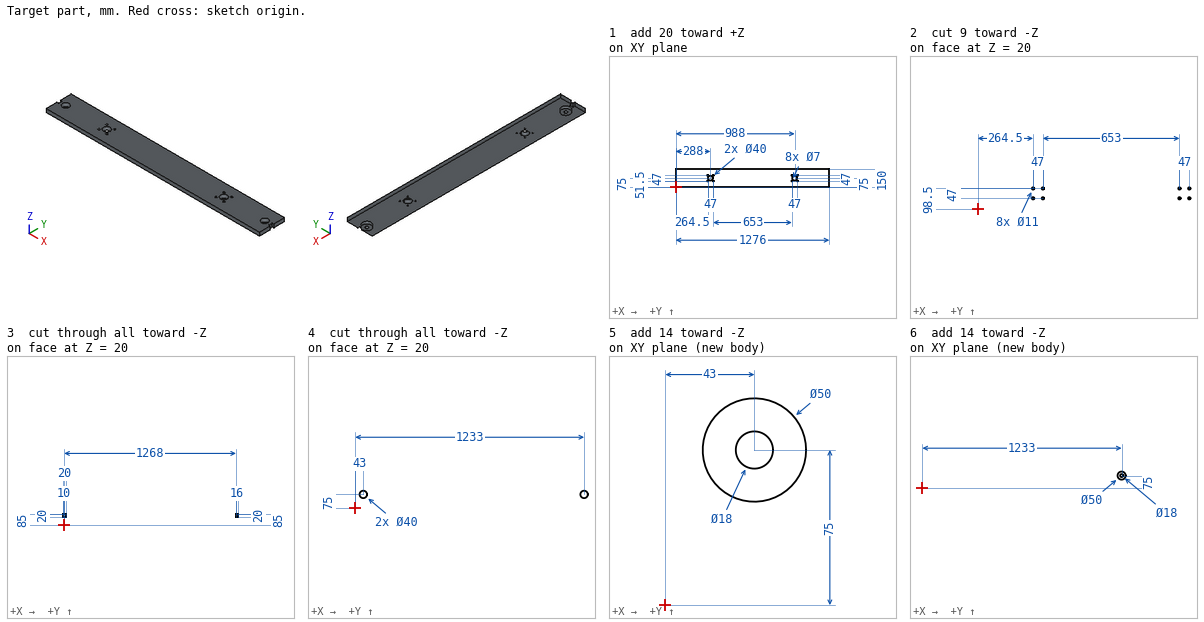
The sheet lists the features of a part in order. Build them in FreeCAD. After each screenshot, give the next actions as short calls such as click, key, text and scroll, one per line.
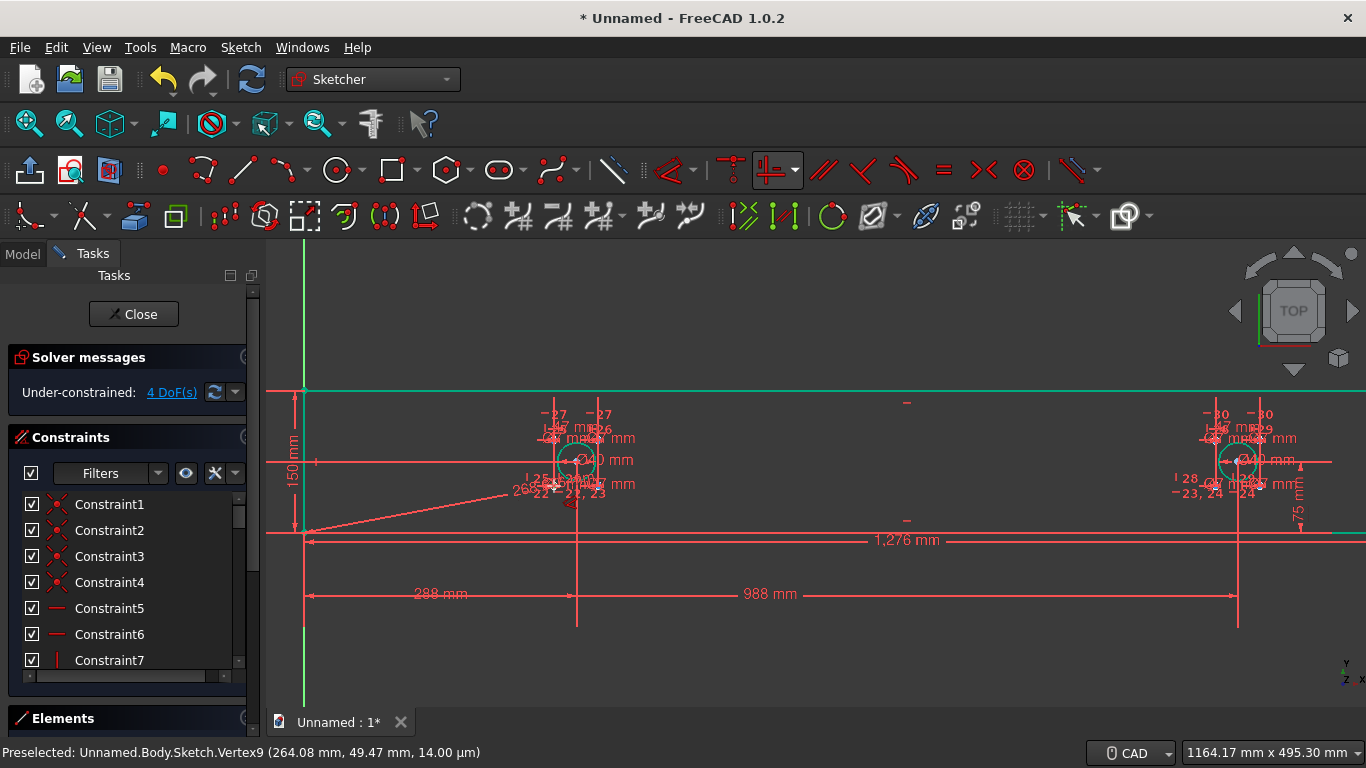
click(554, 440)
click(520, 463)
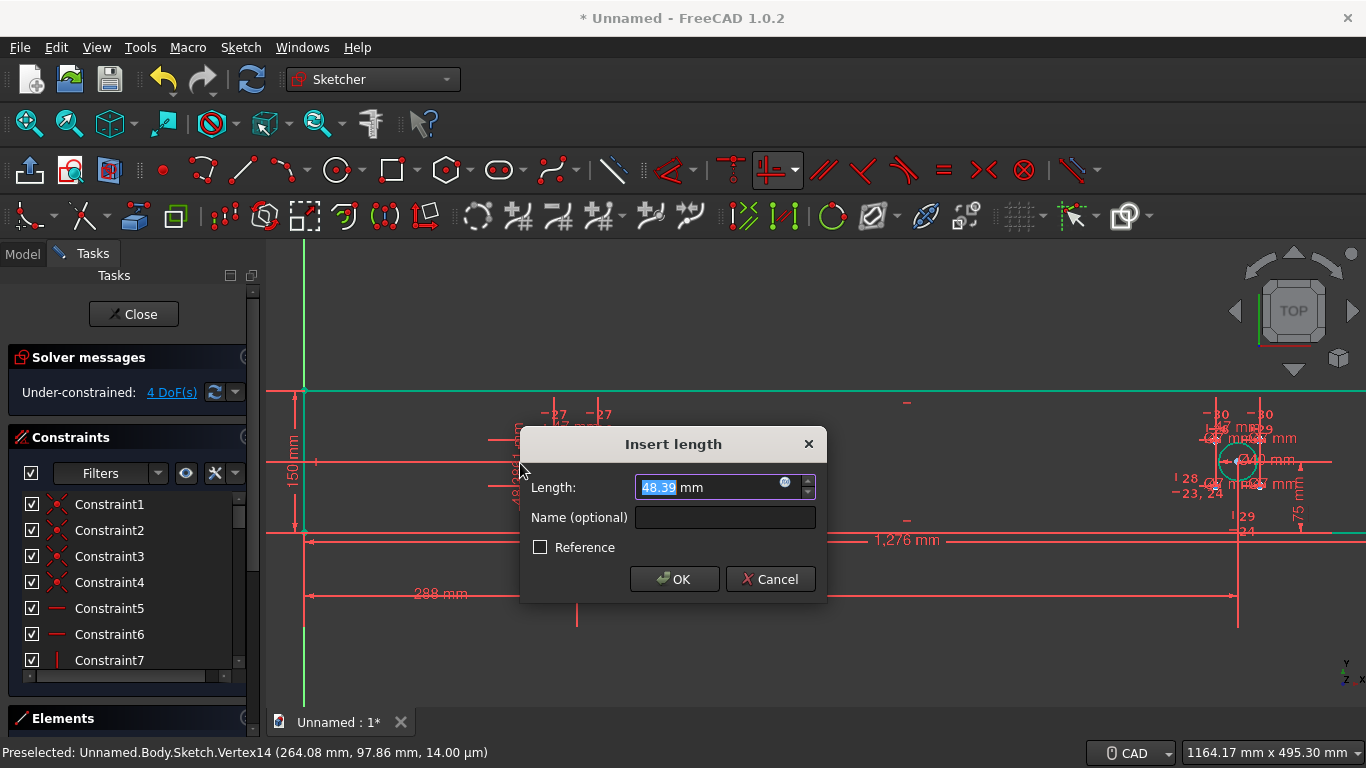
text(47)
key(Return)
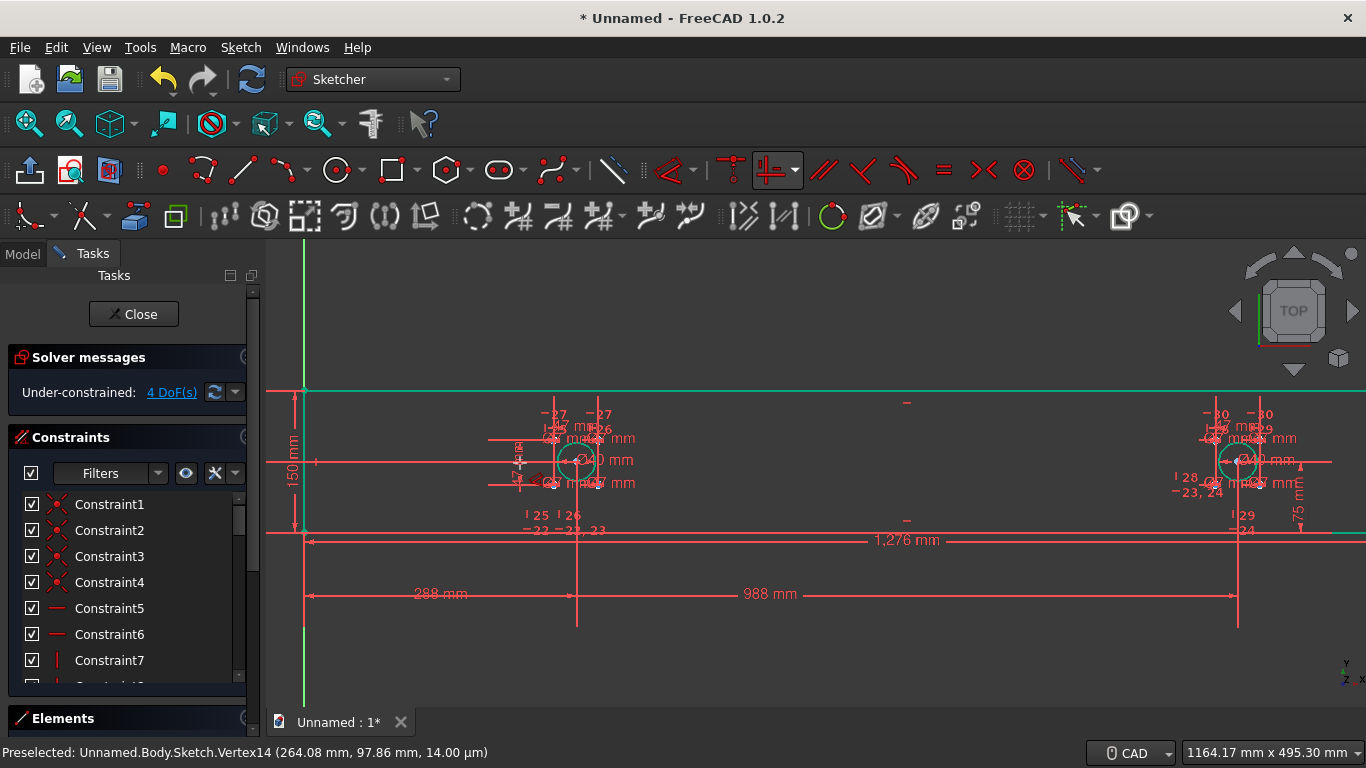
scroll(553, 487, down, 3)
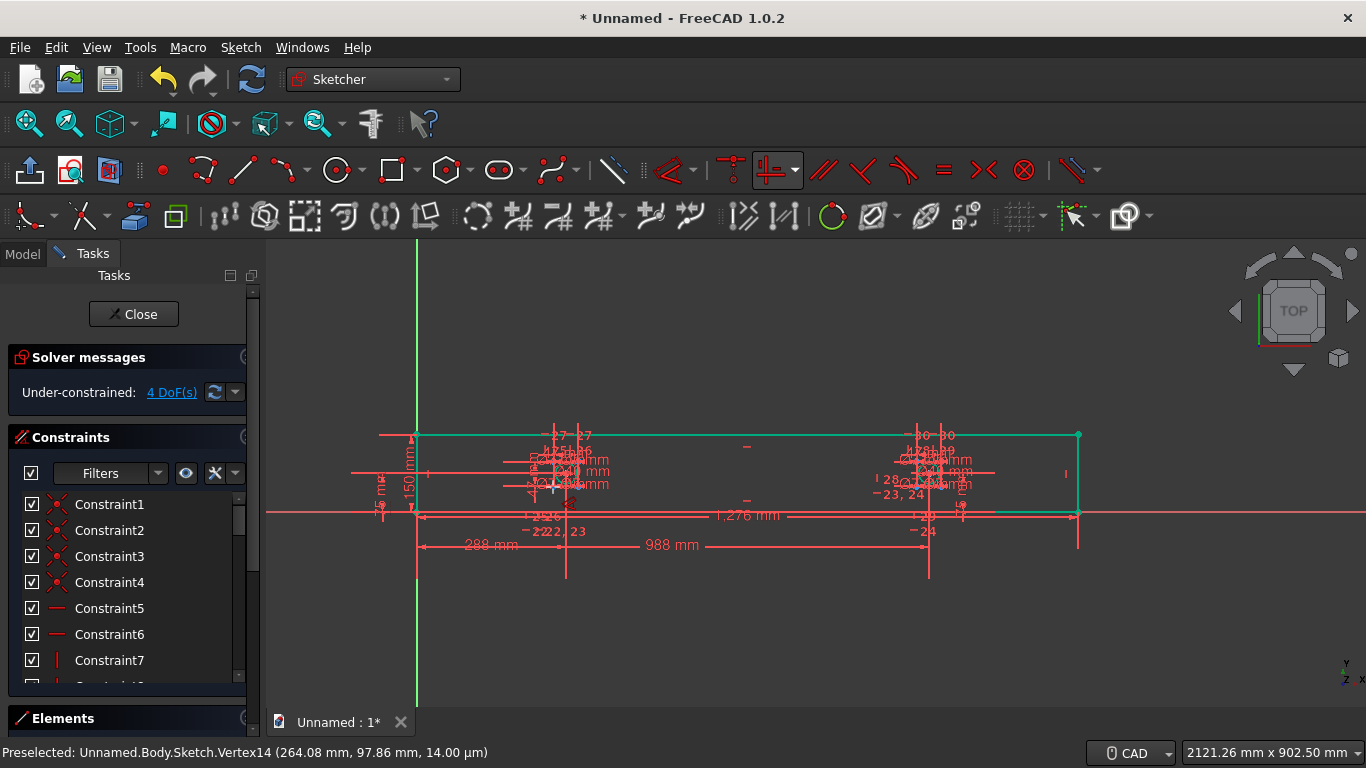
scroll(917, 486, up, 3)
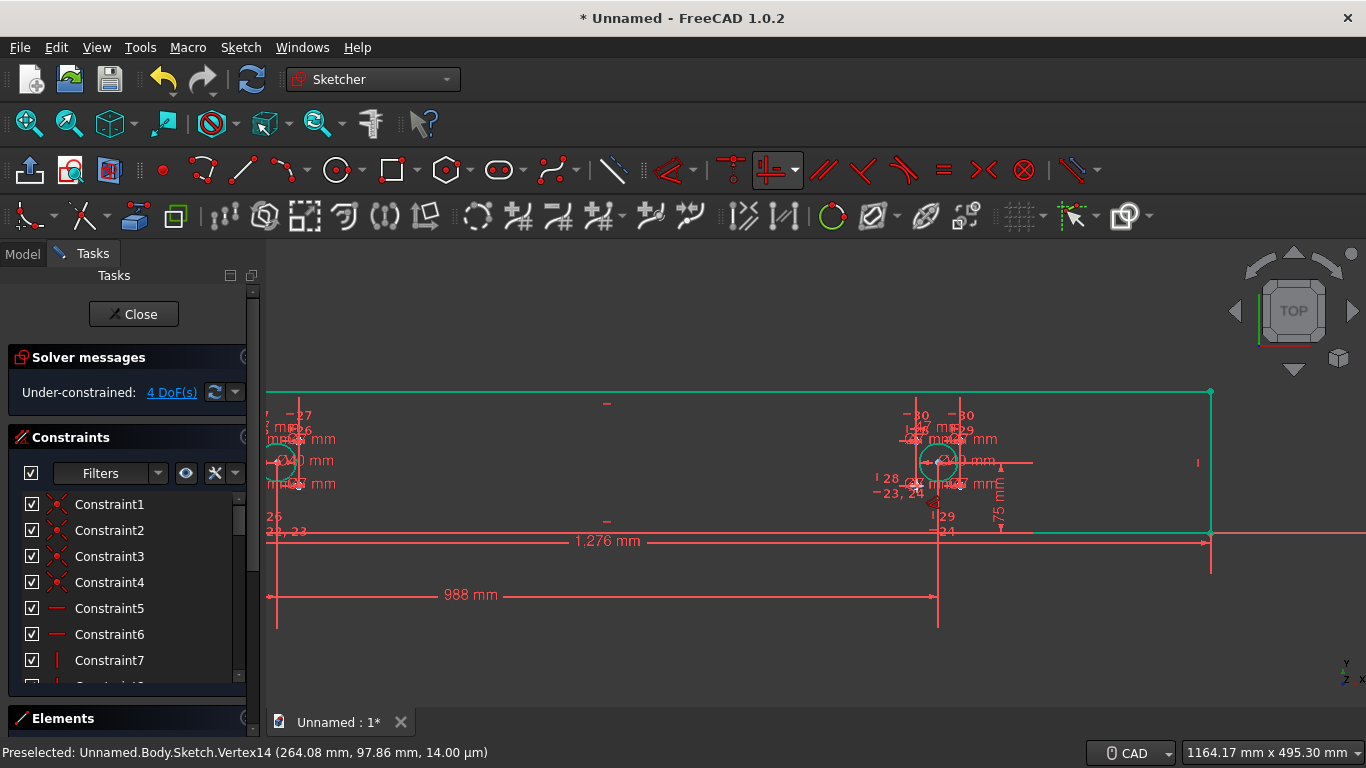
click(916, 486)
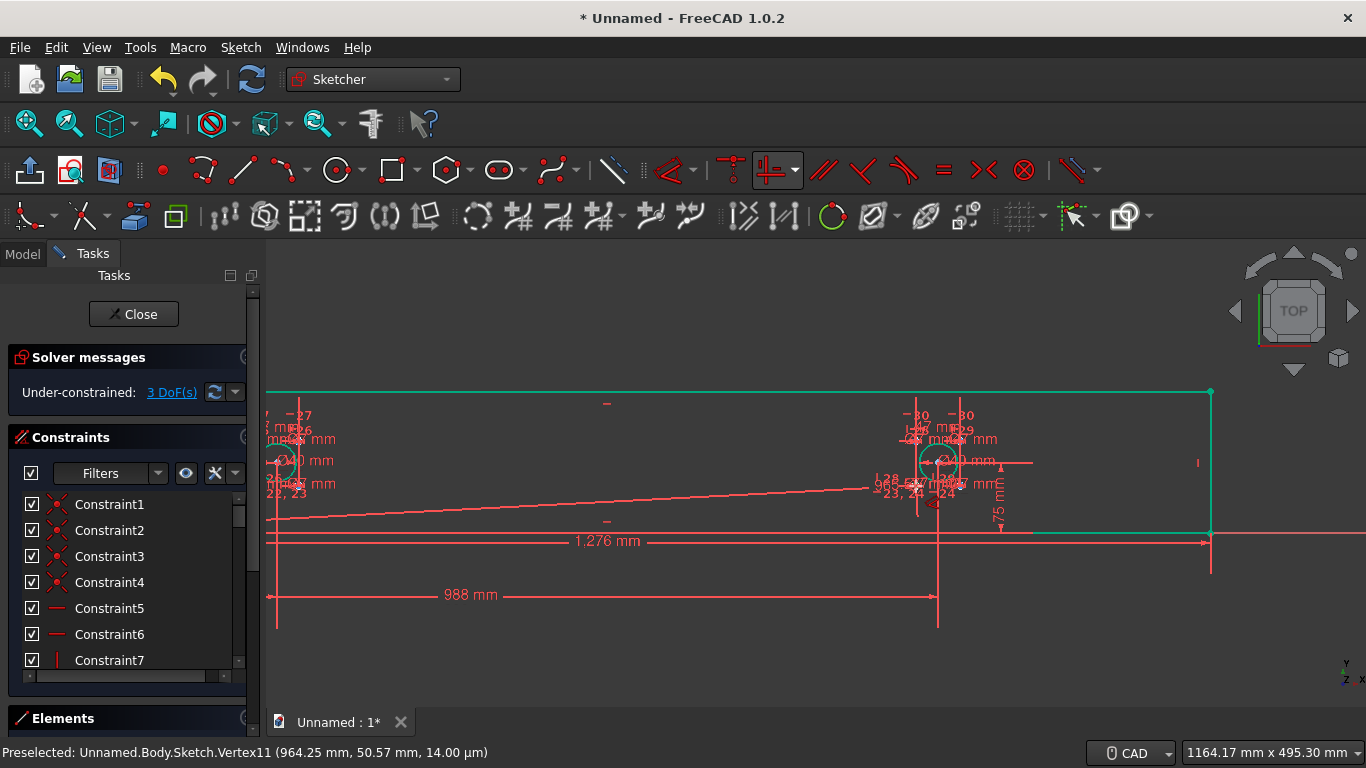
click(916, 441)
click(882, 463)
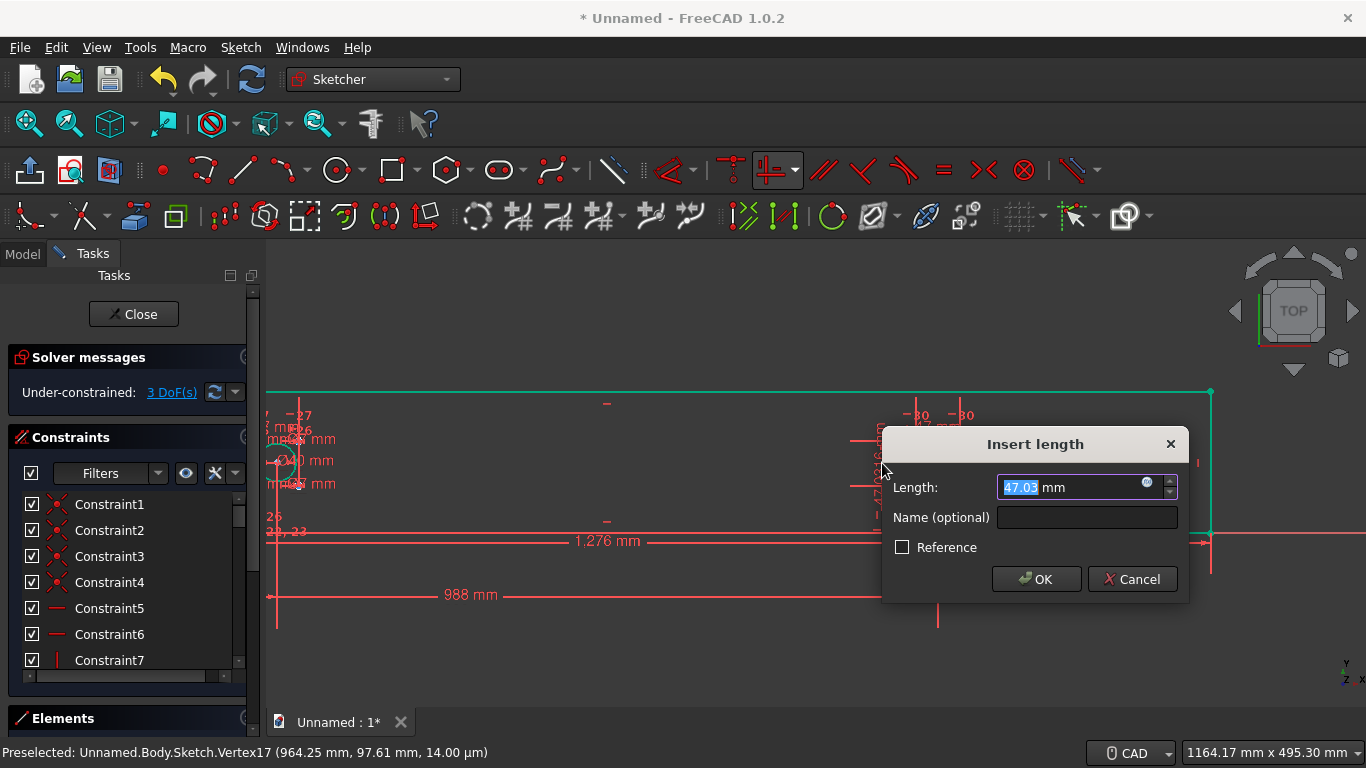
text(47)
key(Return)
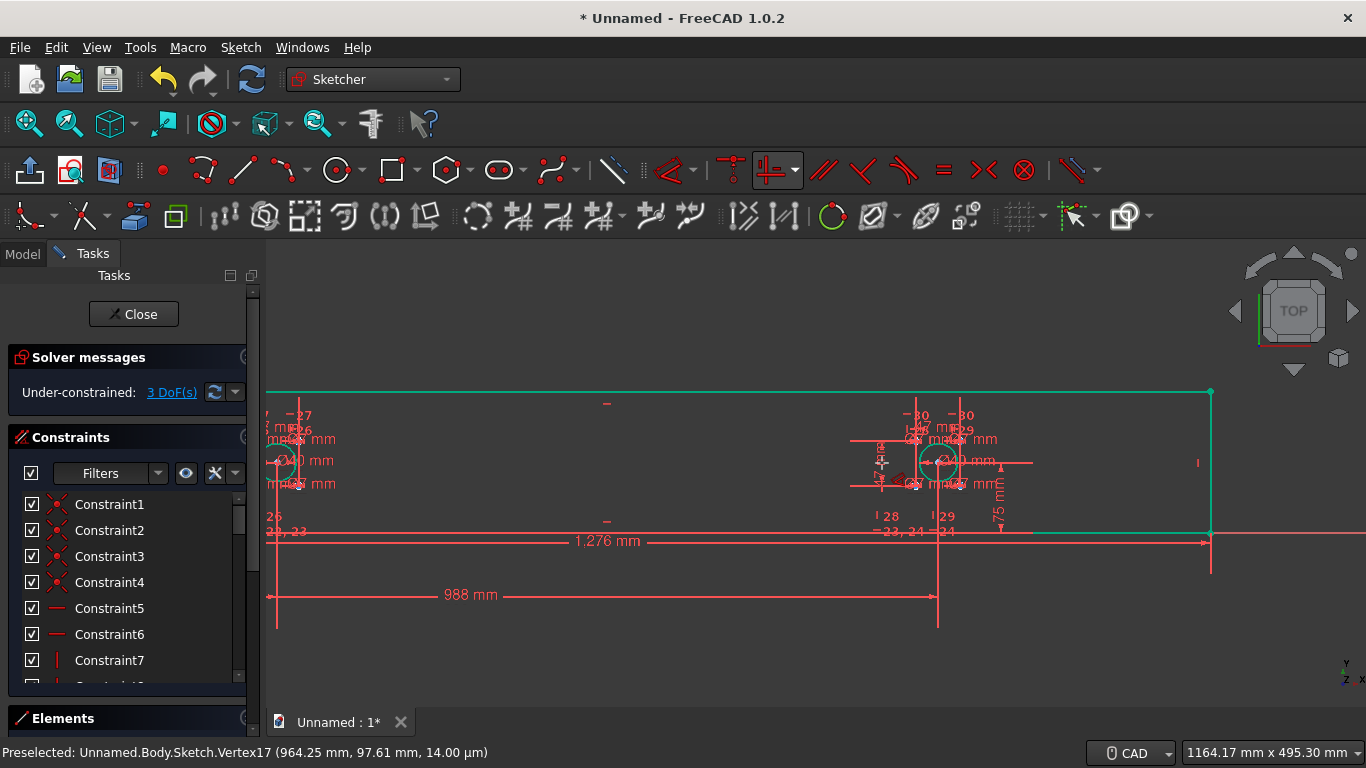
scroll(918, 486, down, 3)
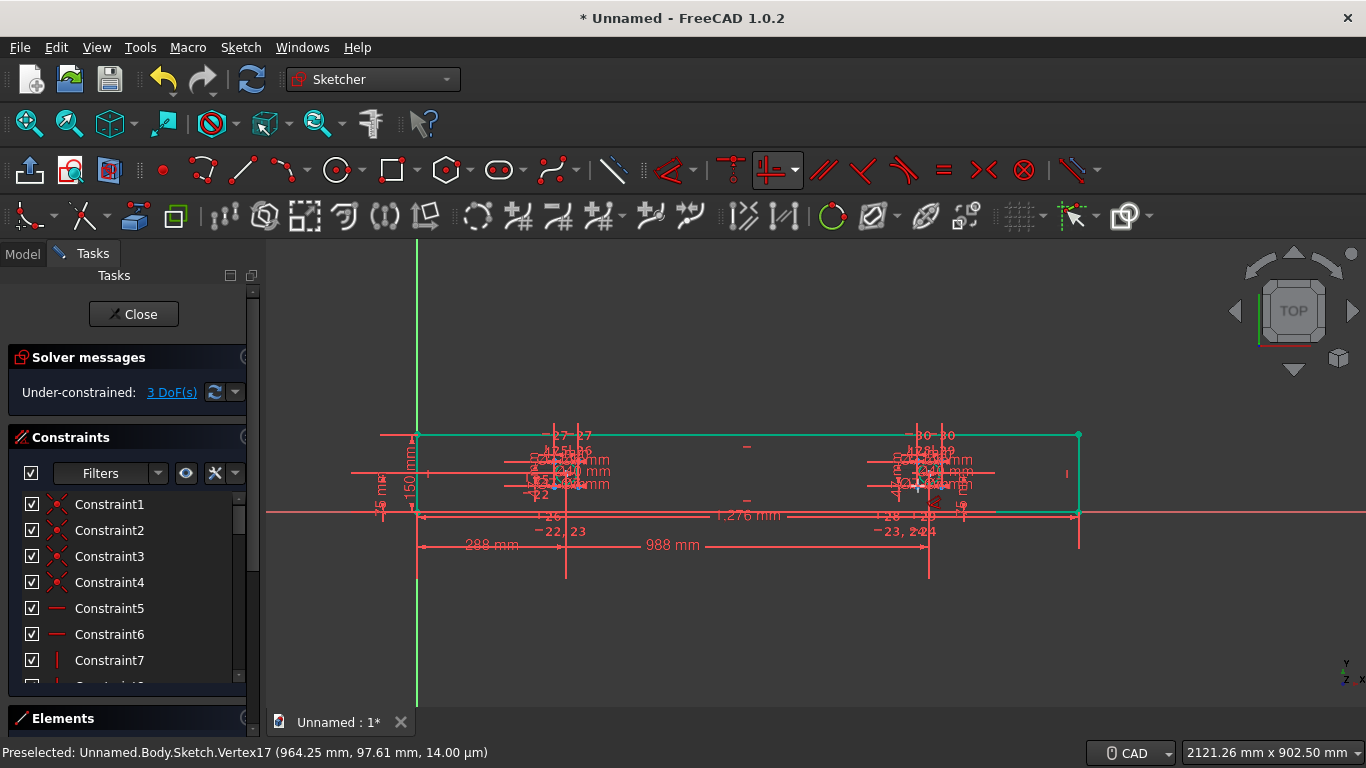
scroll(554, 486, up, 2)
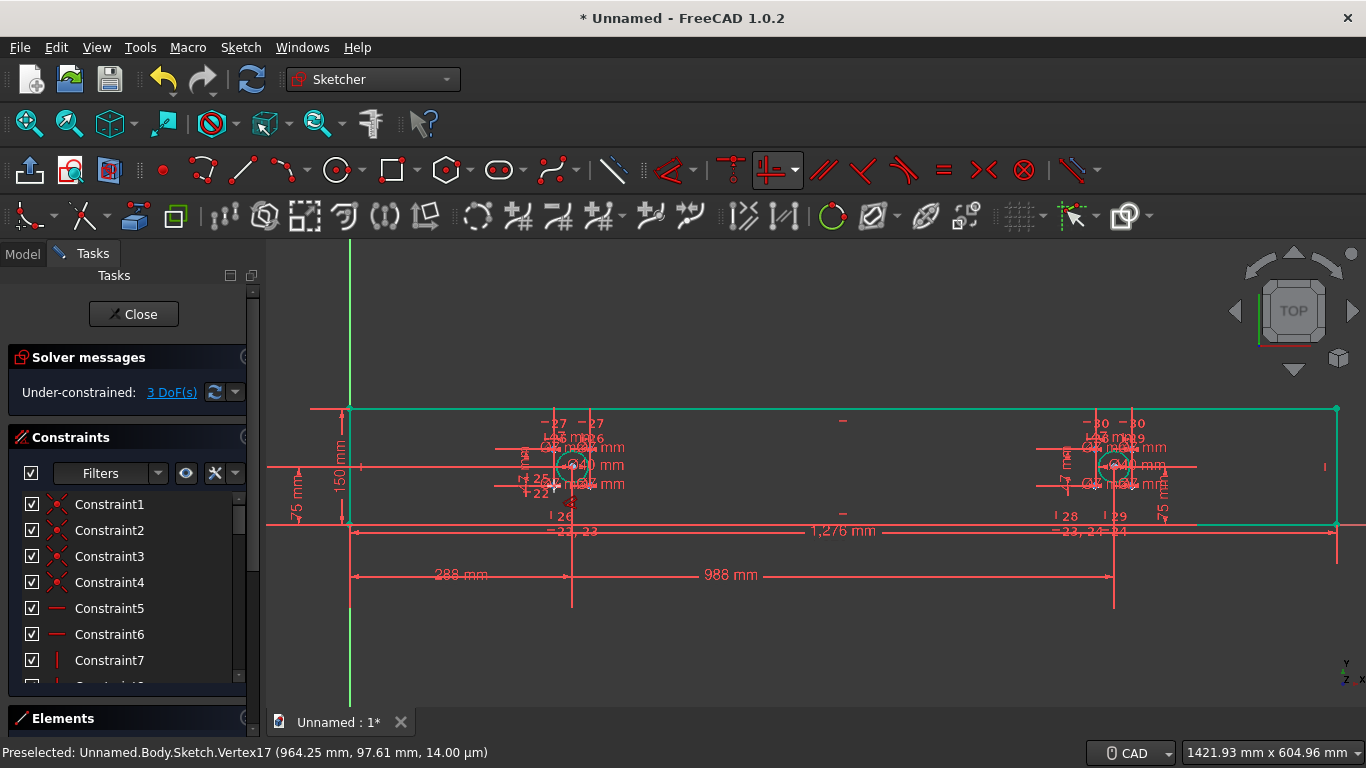
click(554, 486)
click(588, 505)